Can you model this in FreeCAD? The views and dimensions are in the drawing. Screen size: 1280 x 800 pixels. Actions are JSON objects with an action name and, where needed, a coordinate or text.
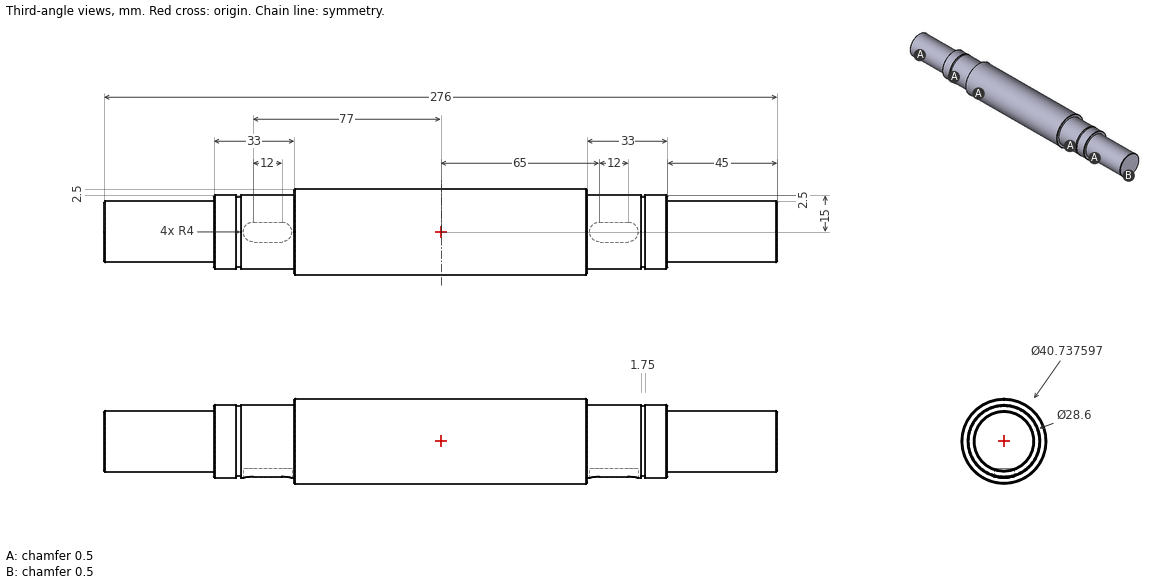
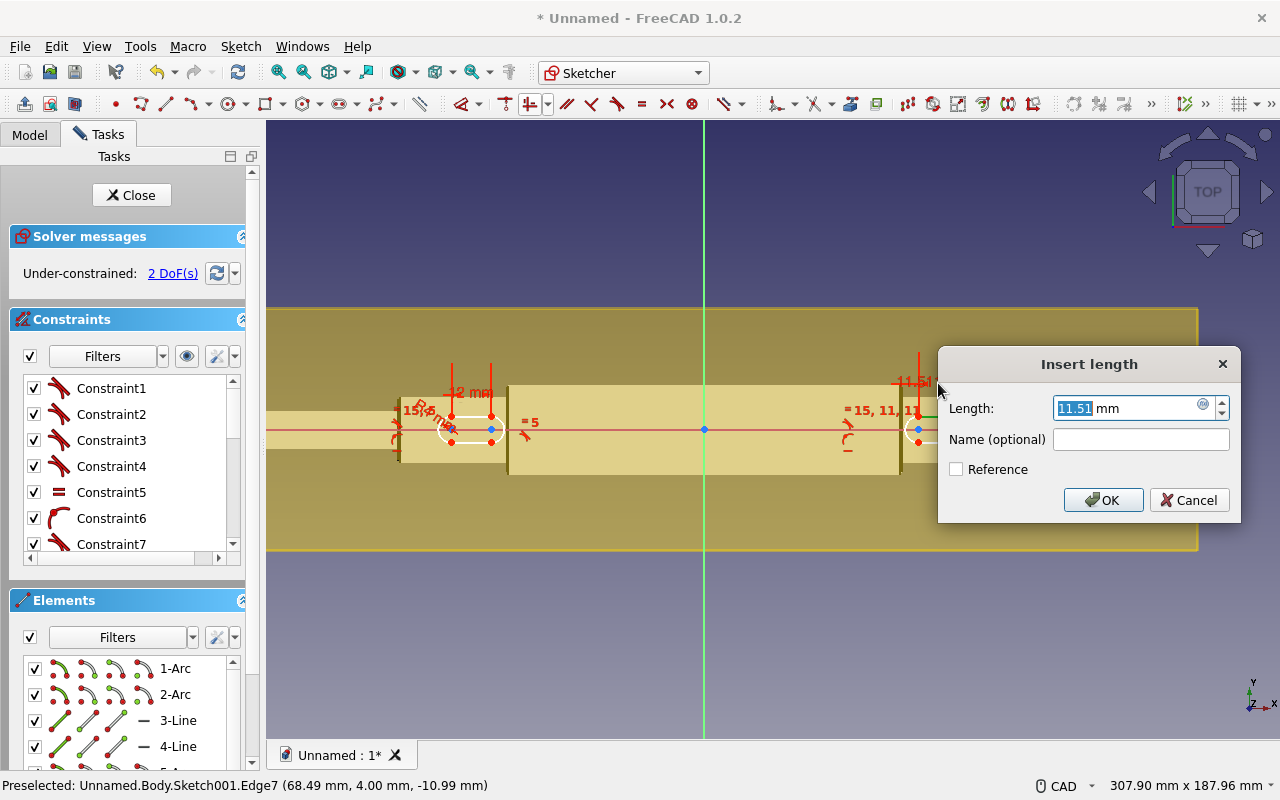
{"action": "type", "text": "12"}
{"action": "key", "text": "Return"}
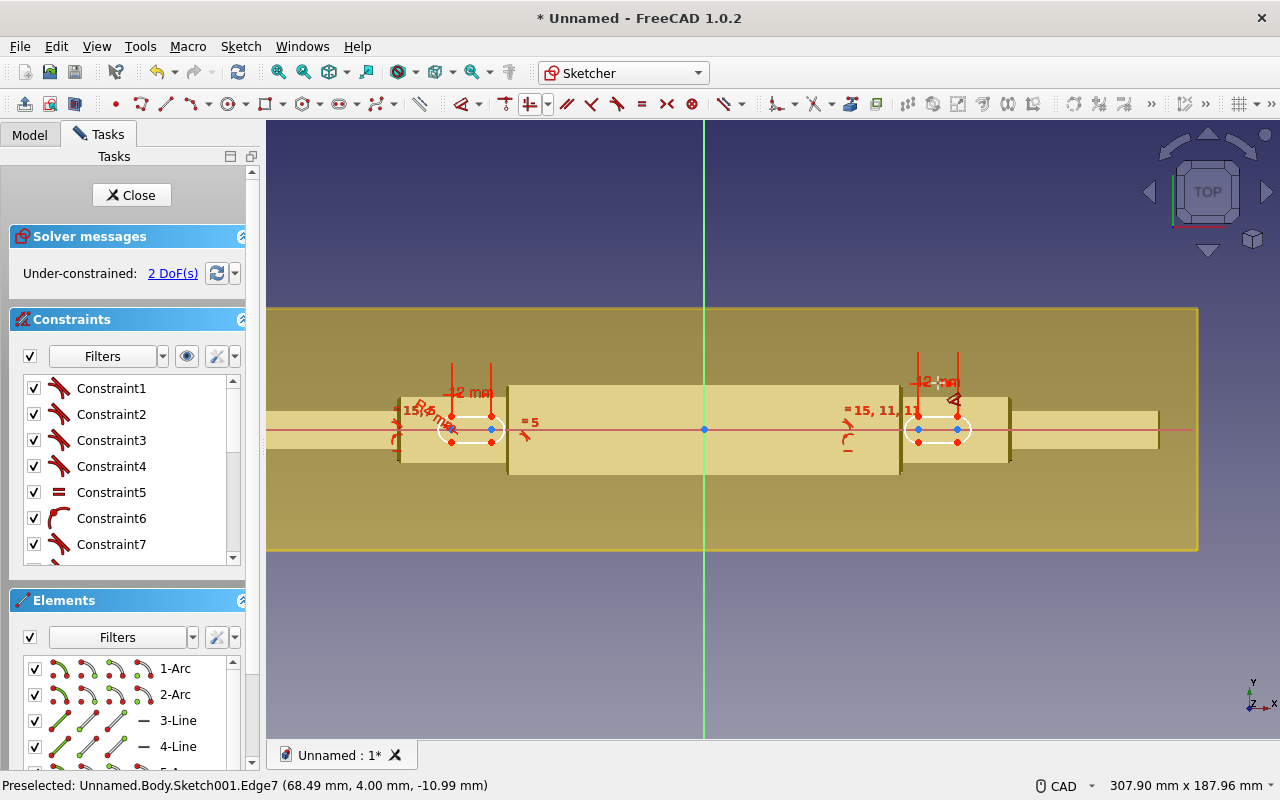
{"action": "left_click", "coordinate": [452, 417]}
{"action": "left_click", "coordinate": [578, 383]}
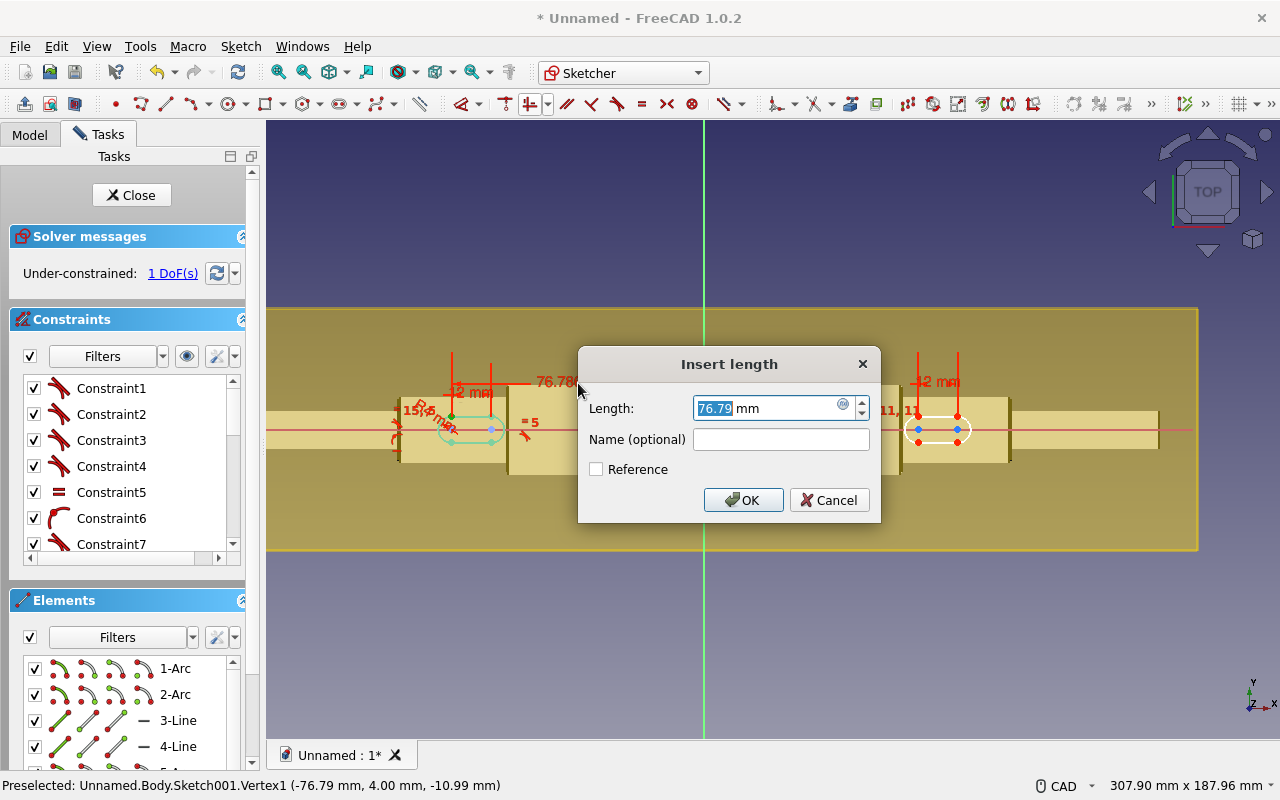
{"action": "type", "text": "77"}
{"action": "key", "text": "Return"}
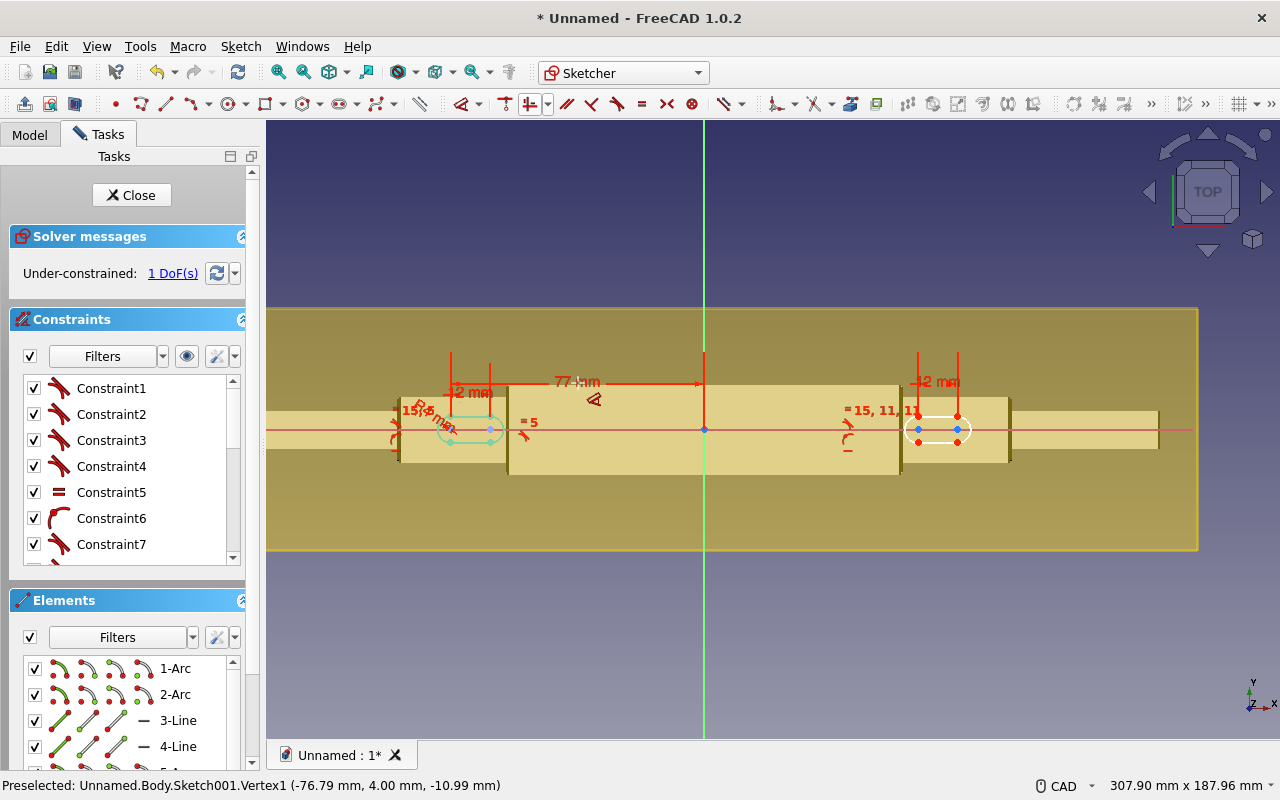
{"action": "left_click", "coordinate": [918, 417]}
{"action": "left_click", "coordinate": [811, 383]}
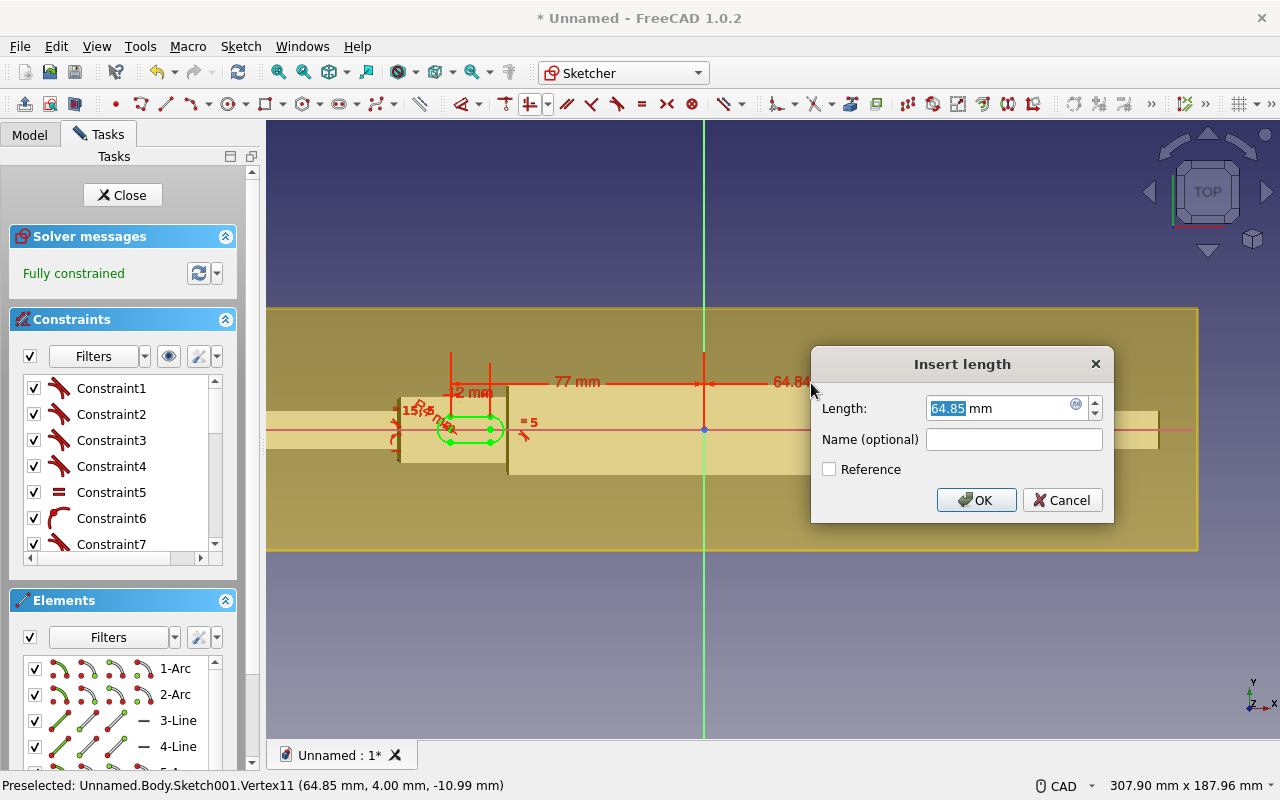
{"action": "type", "text": "65"}
{"action": "key", "text": "Return"}
{"action": "key", "text": "Escape"}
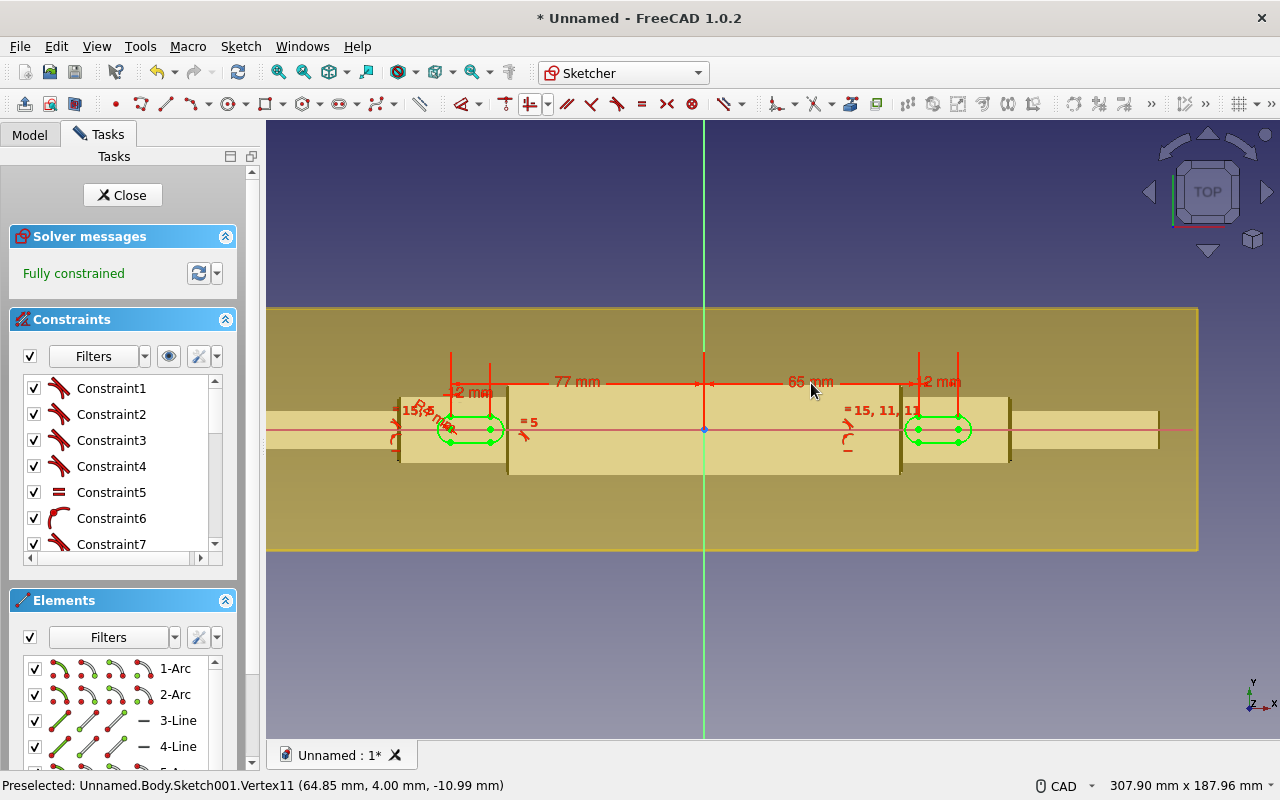
{"action": "left_click", "coordinate": [123, 195]}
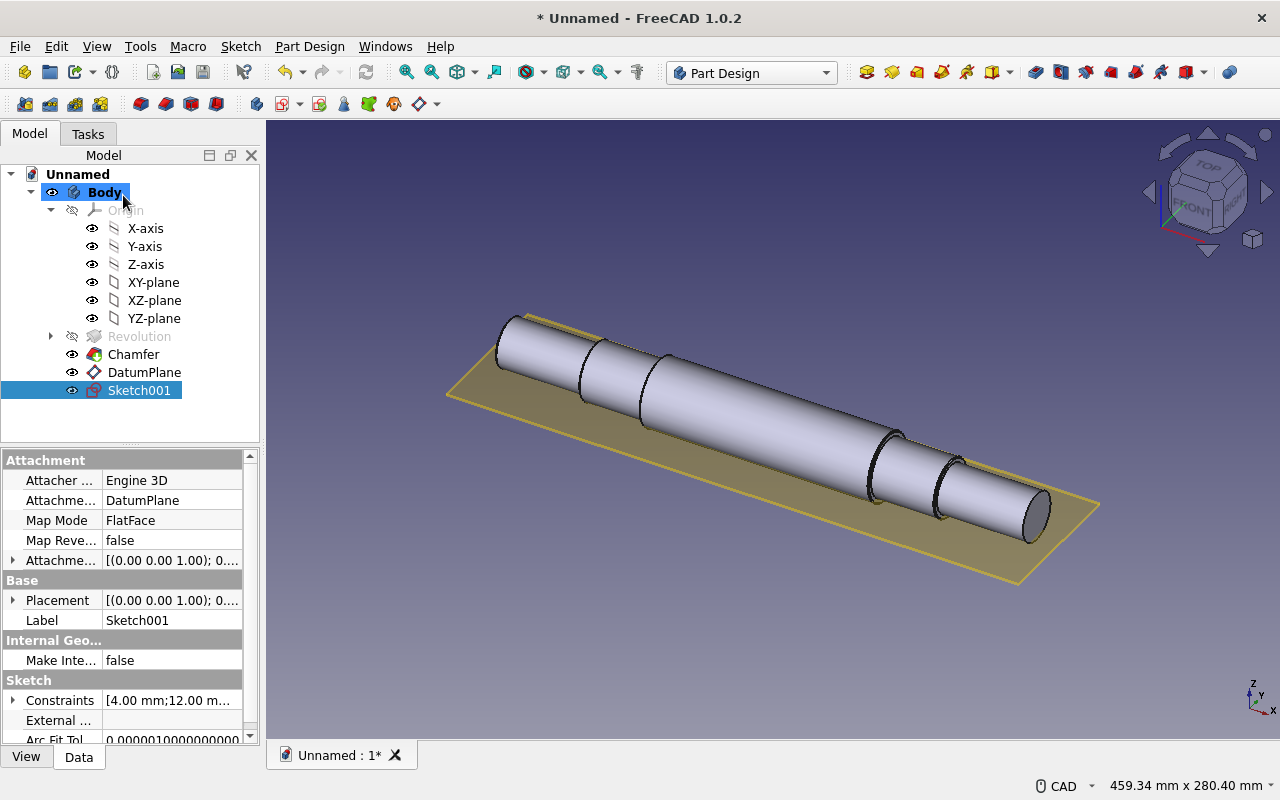
{"action": "left_click", "coordinate": [1036, 72]}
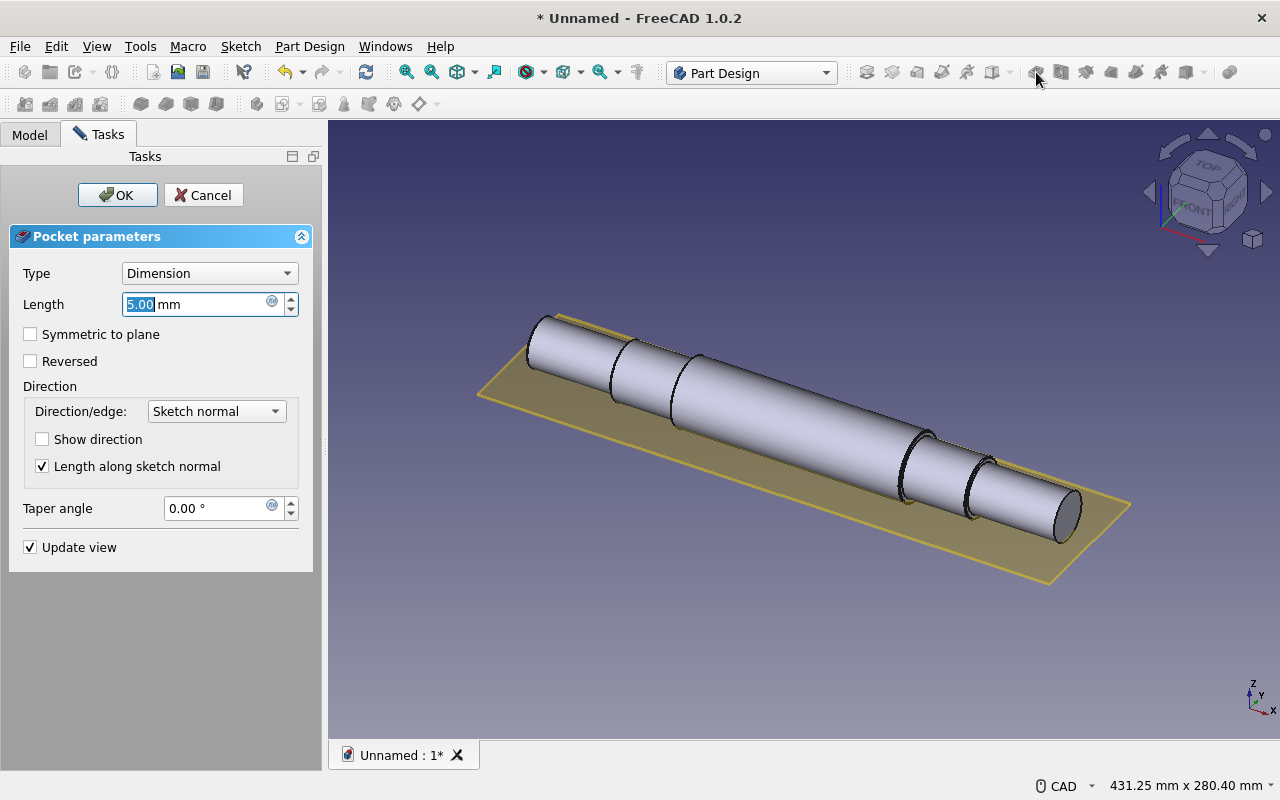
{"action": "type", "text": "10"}
{"action": "key", "text": "Tab"}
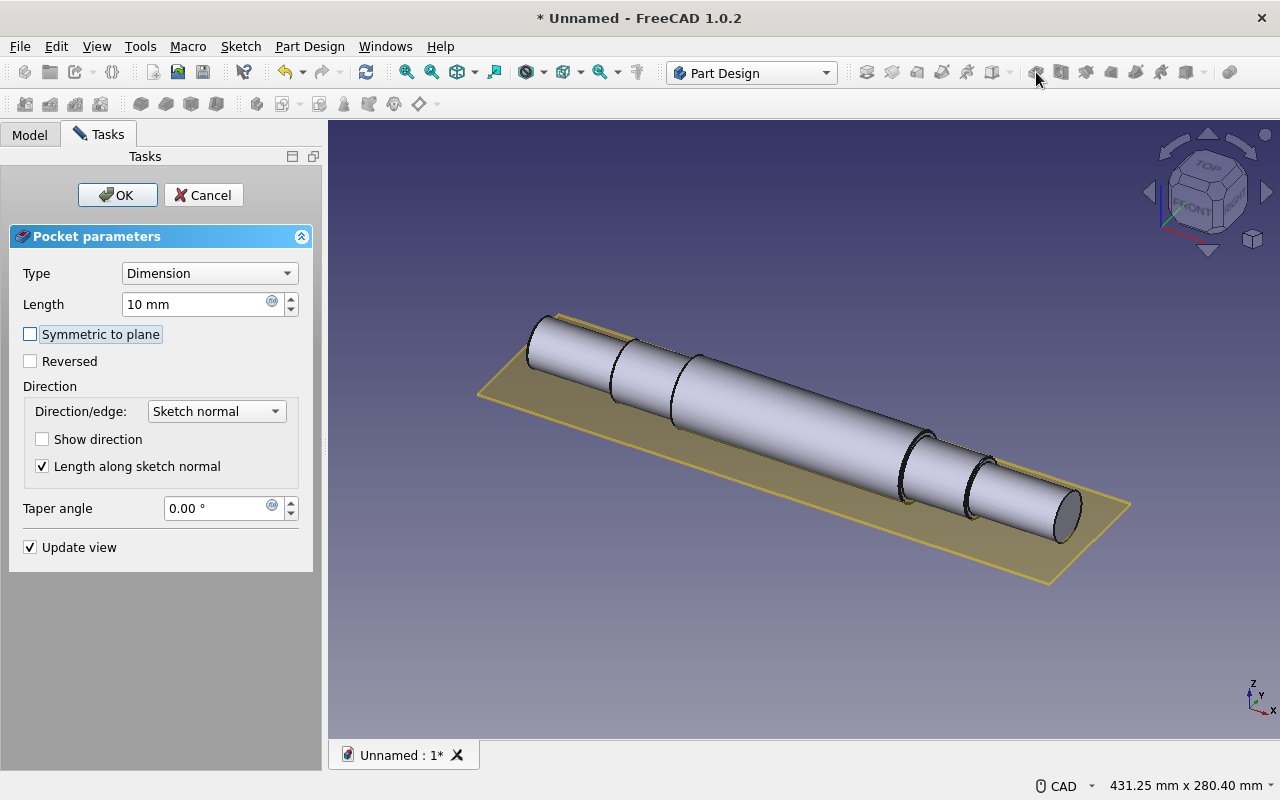
{"action": "left_click", "coordinate": [118, 195]}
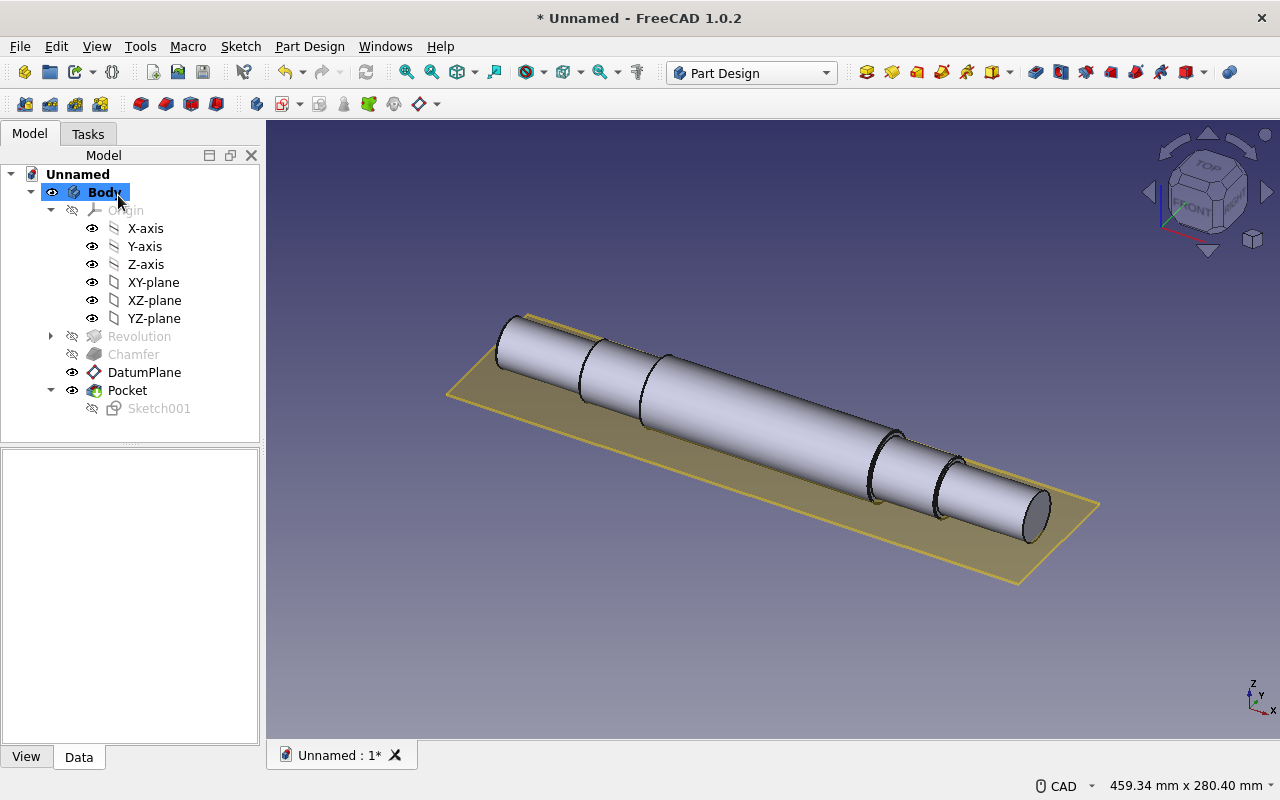
{"action": "left_click", "coordinate": [117, 372]}
{"action": "key", "text": "space"}